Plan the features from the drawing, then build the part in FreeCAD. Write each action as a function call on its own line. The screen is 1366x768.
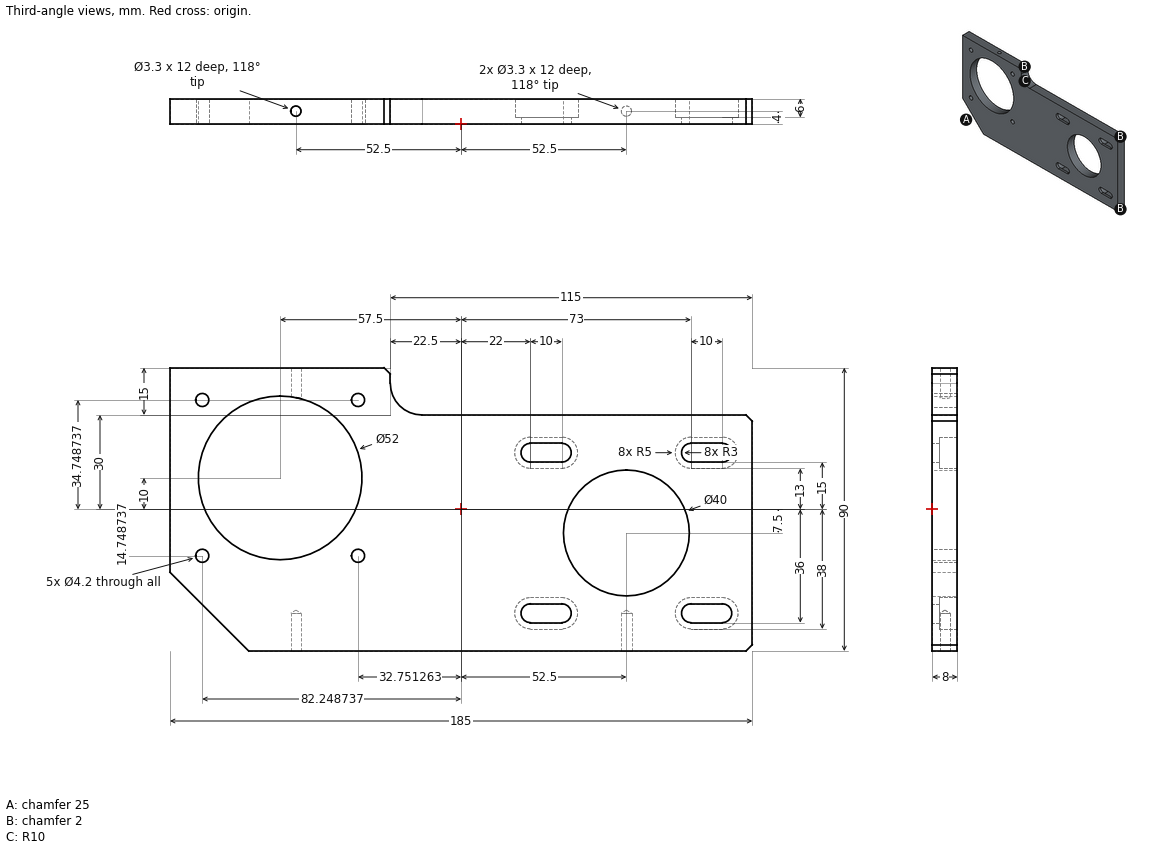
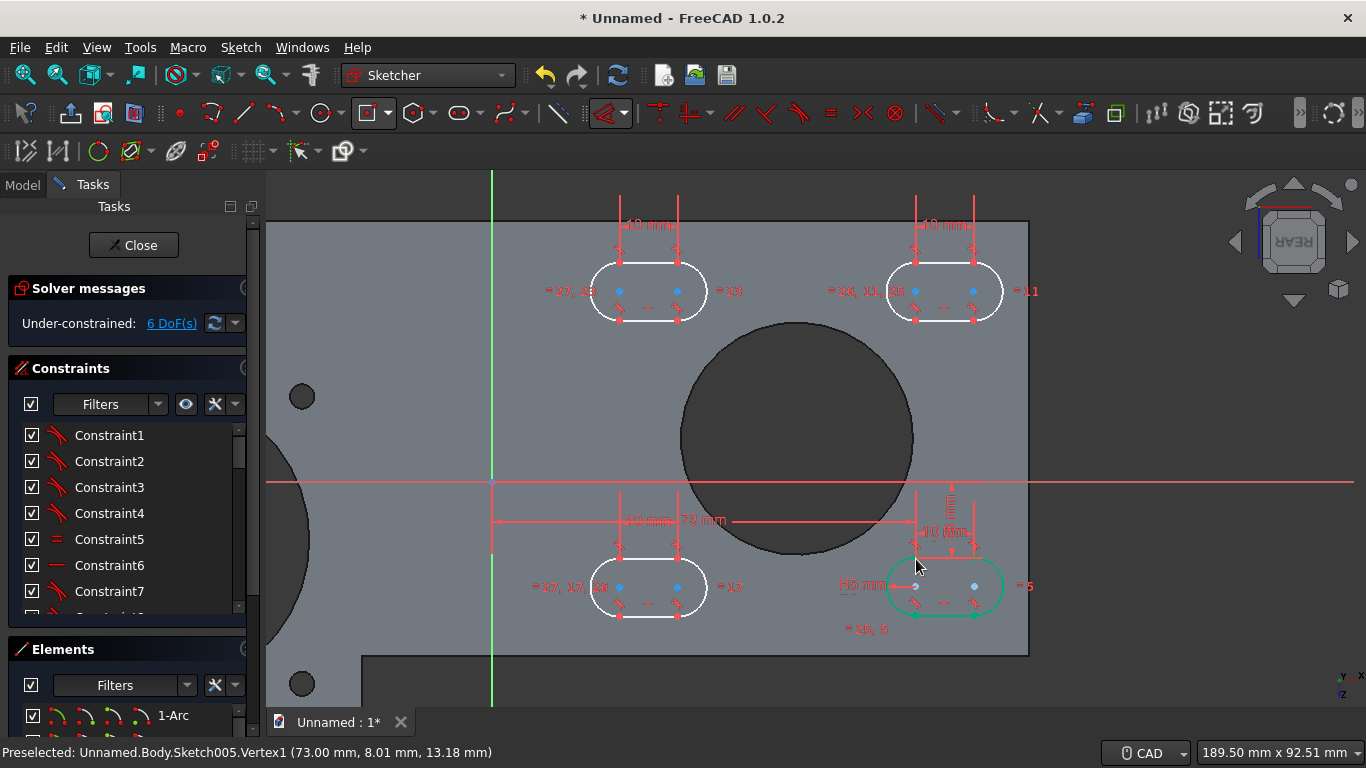
click(916, 263)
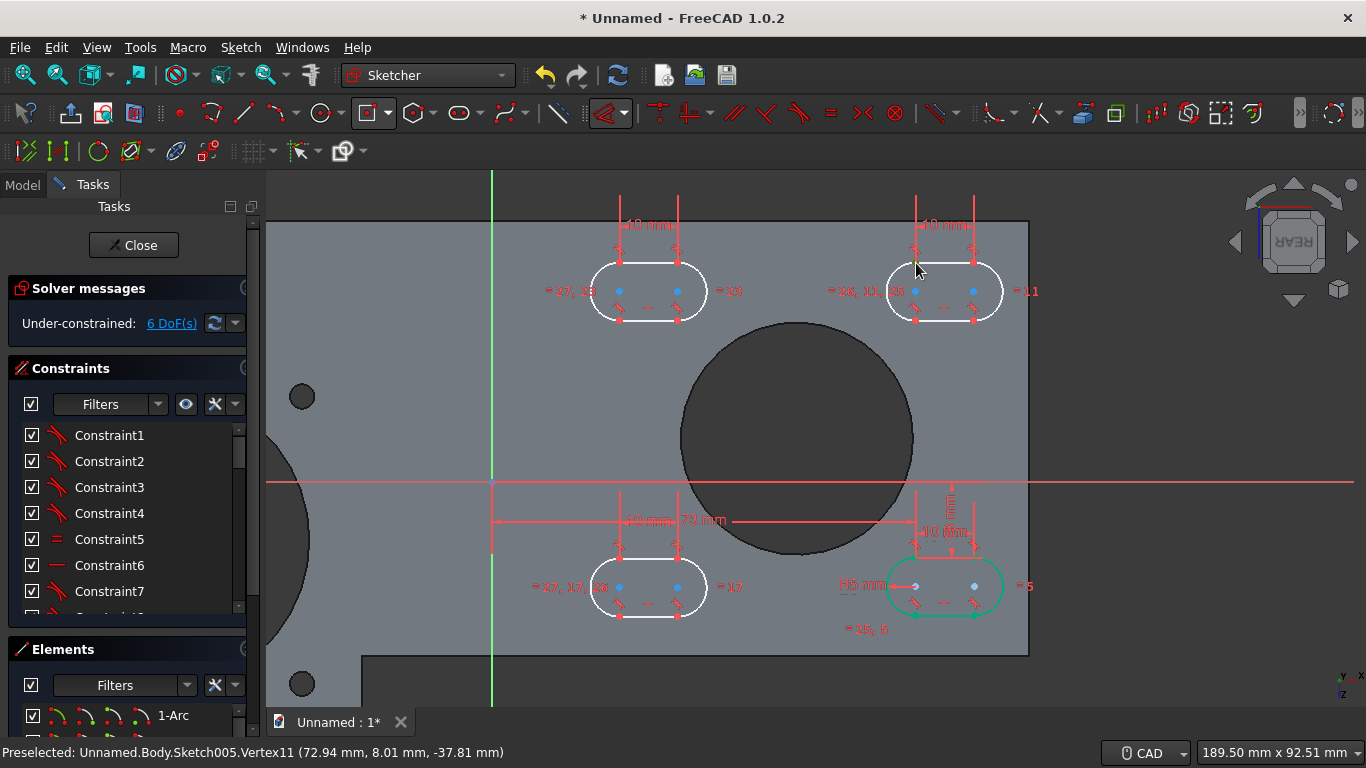
click(626, 114)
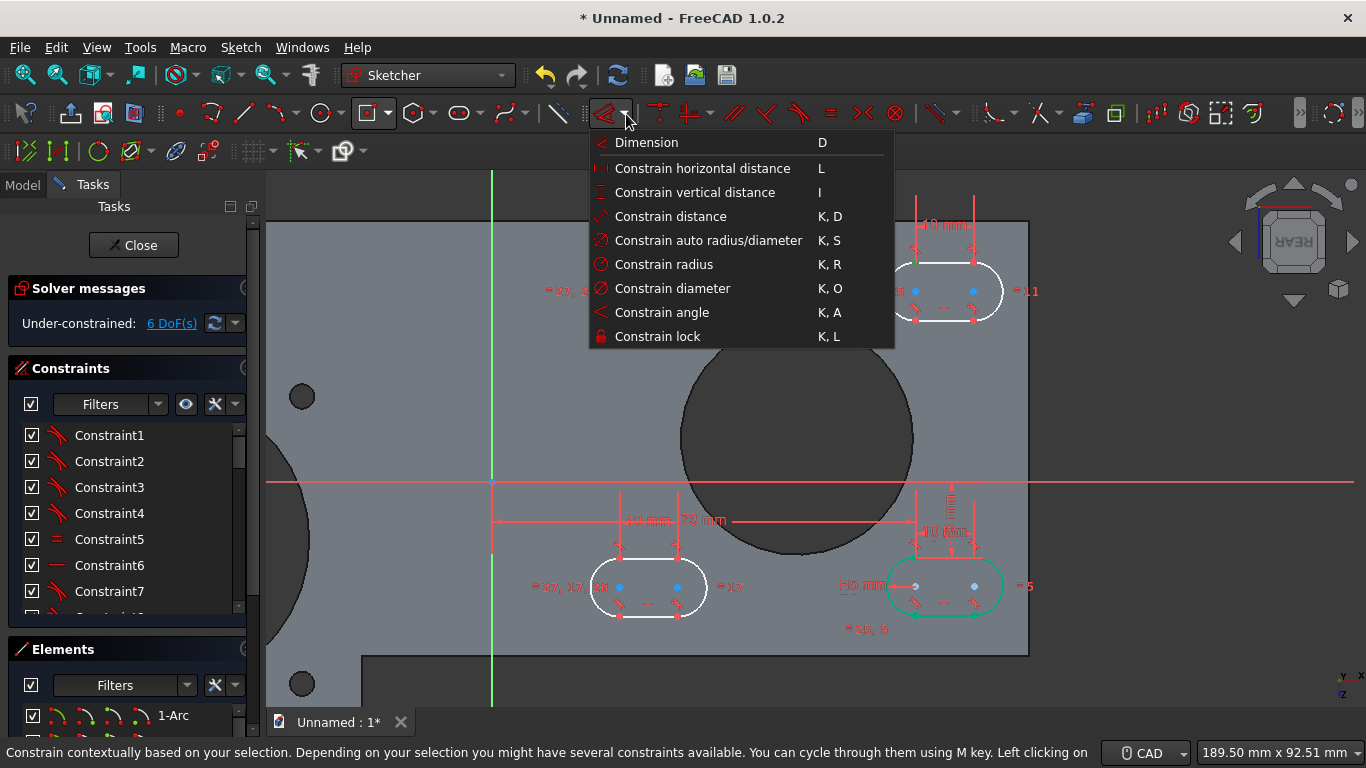
click(742, 168)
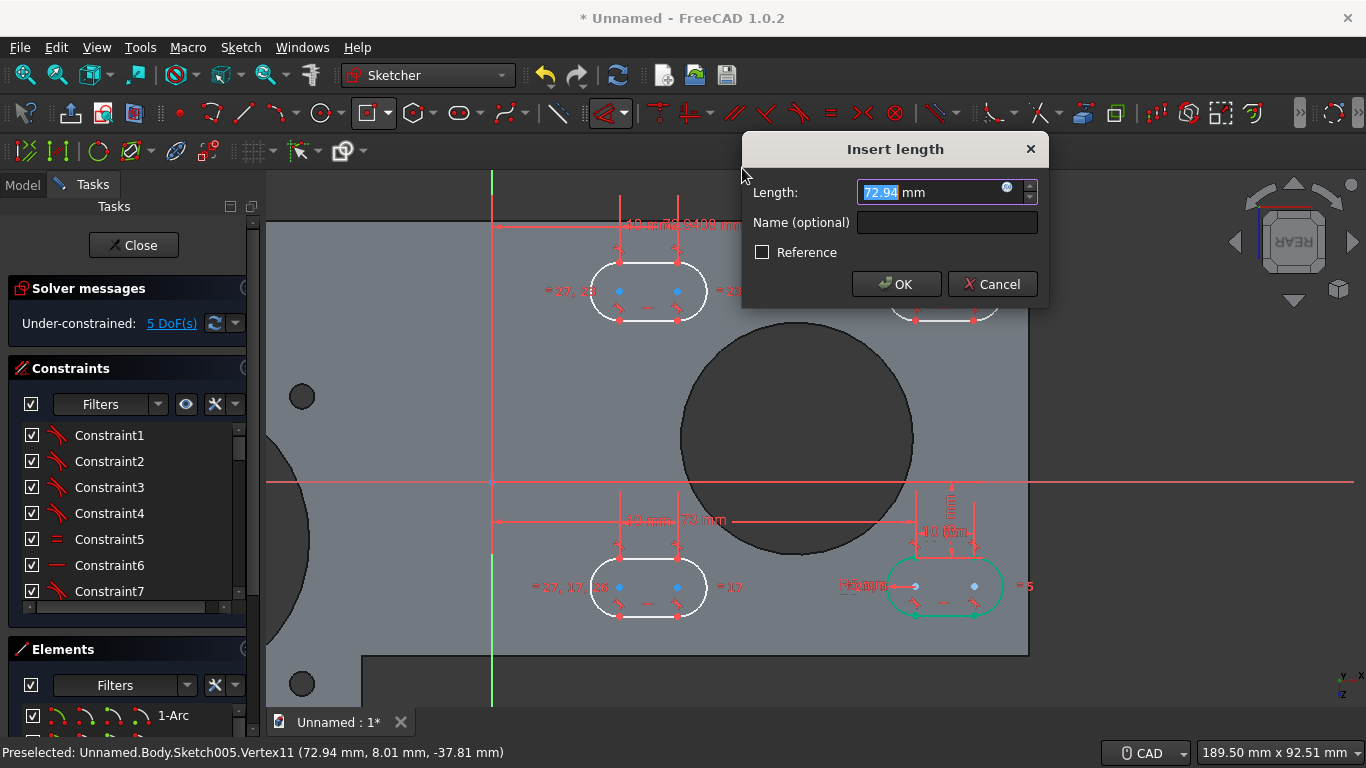
text(73)
key(Return)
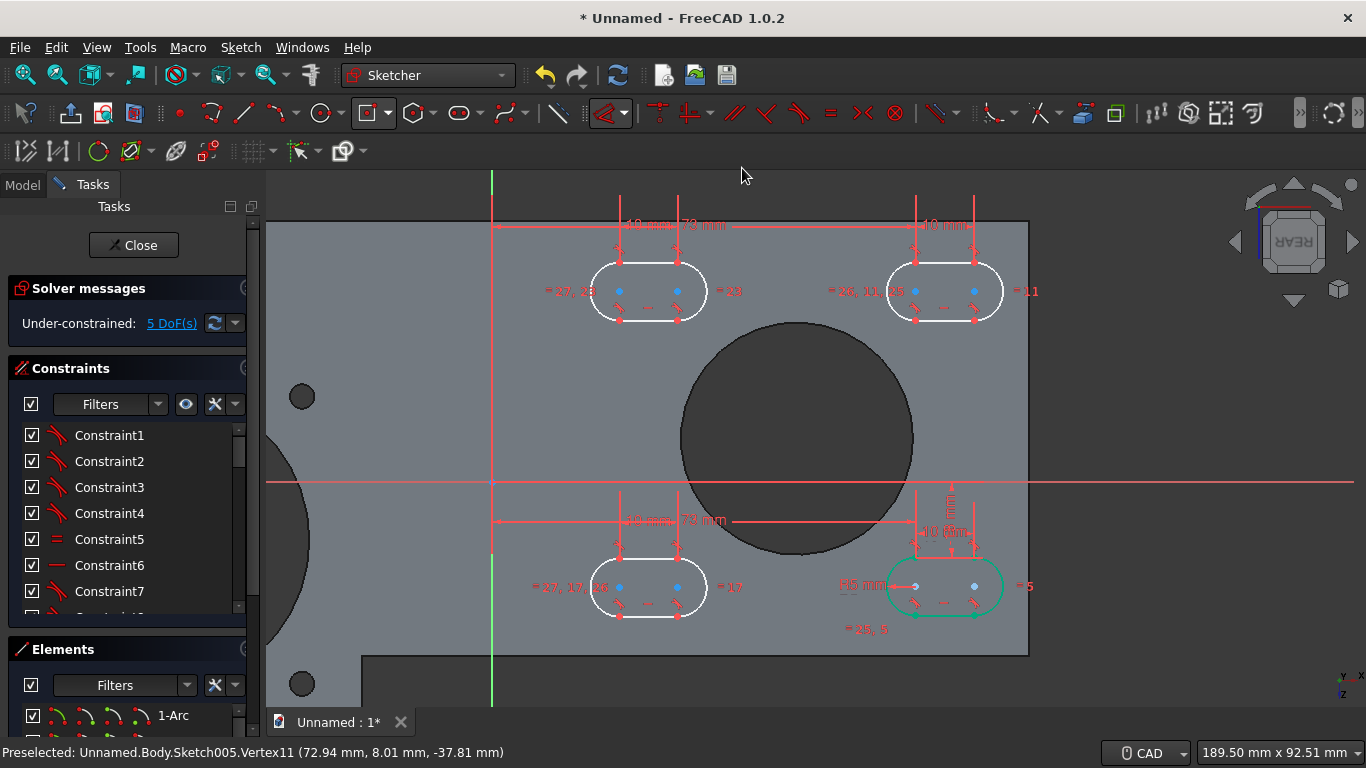
click(916, 263)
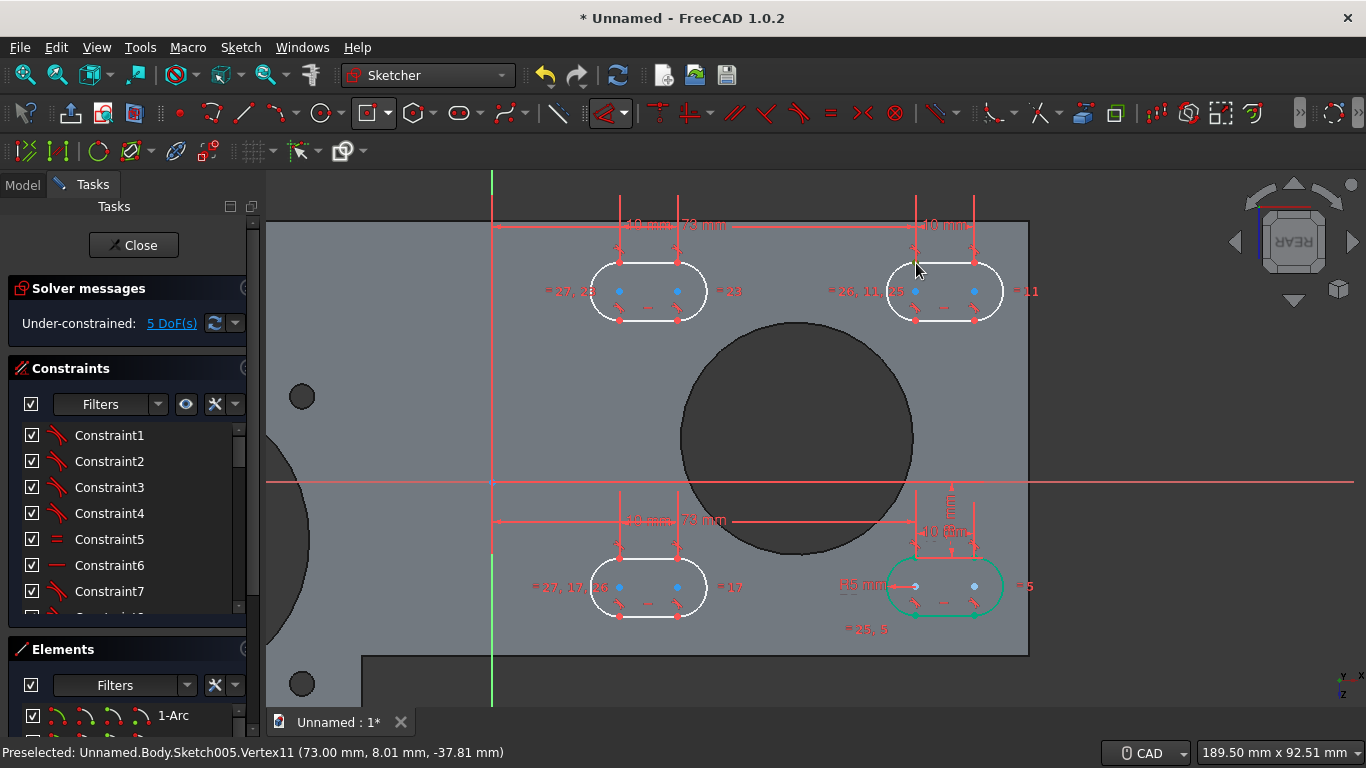
key(i)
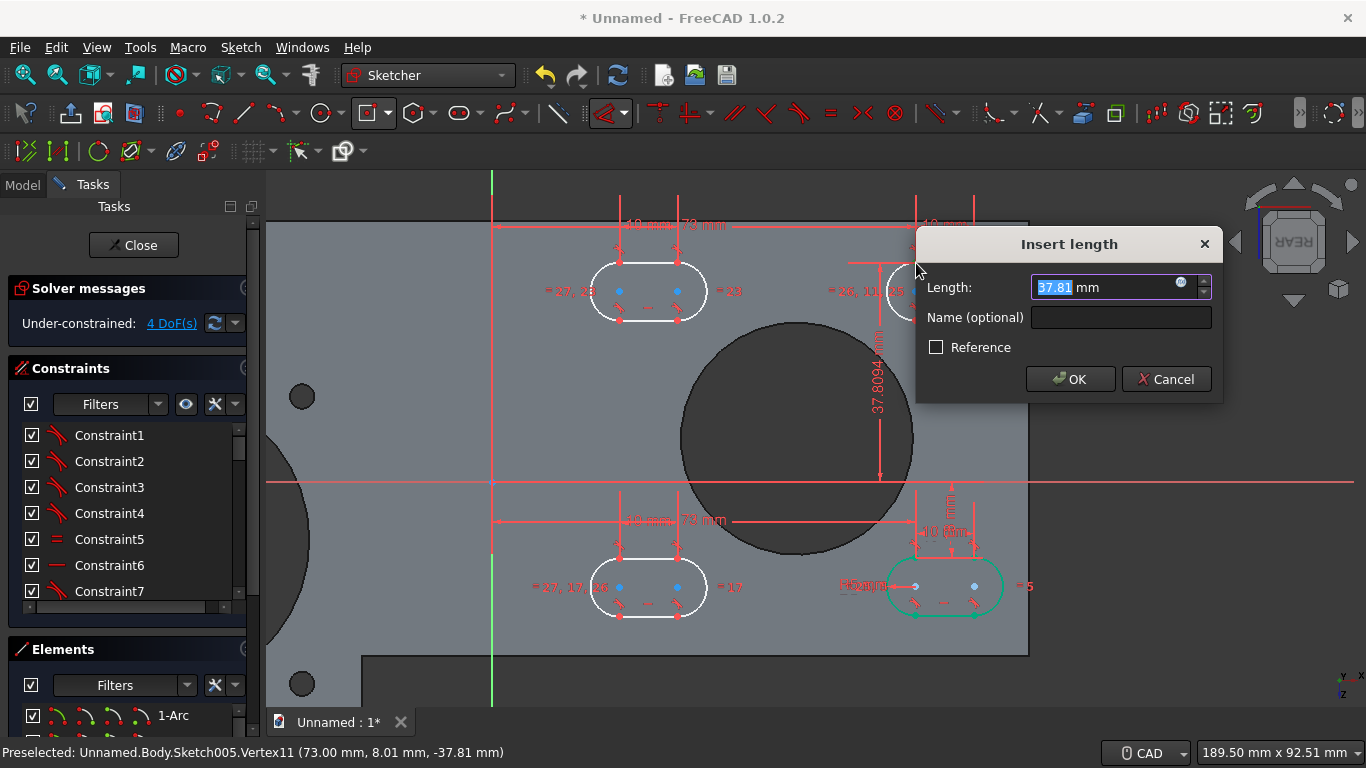
text(38)
key(Return)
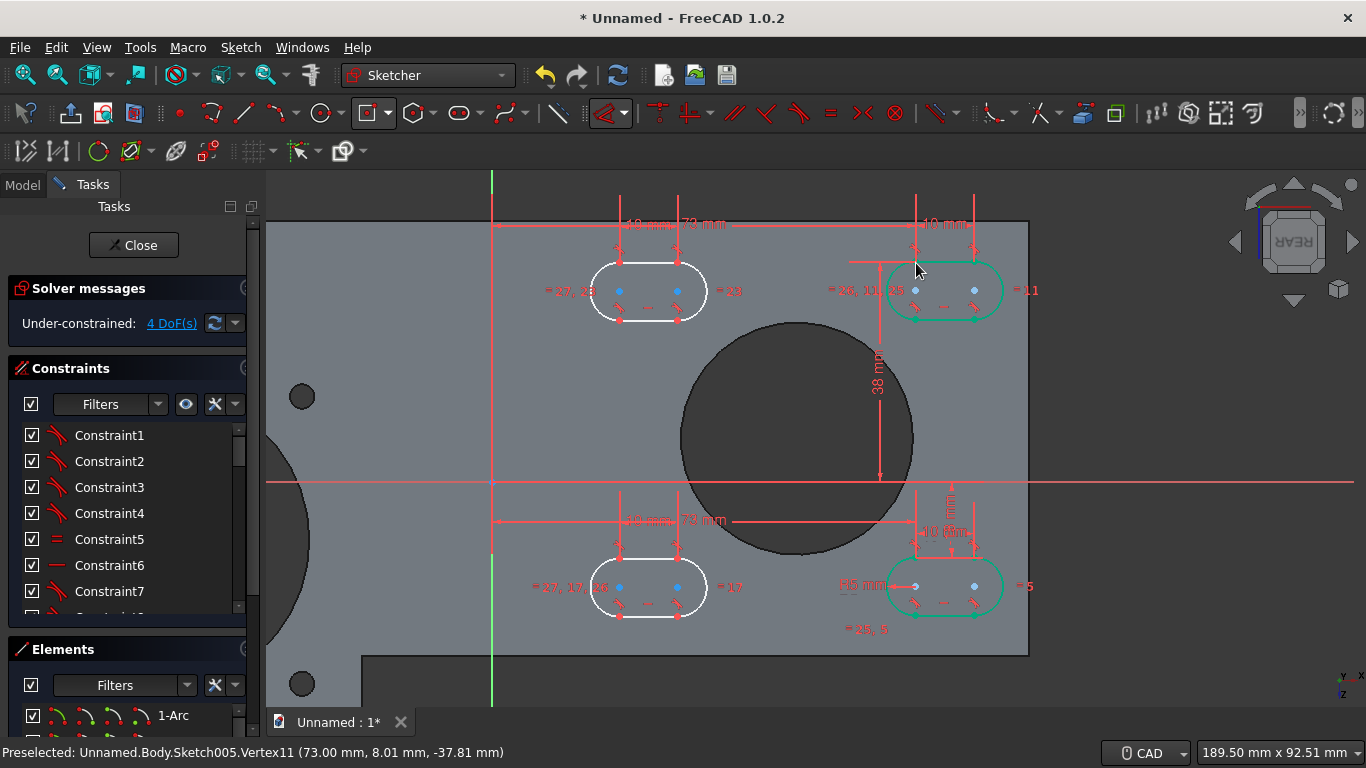
click(620, 559)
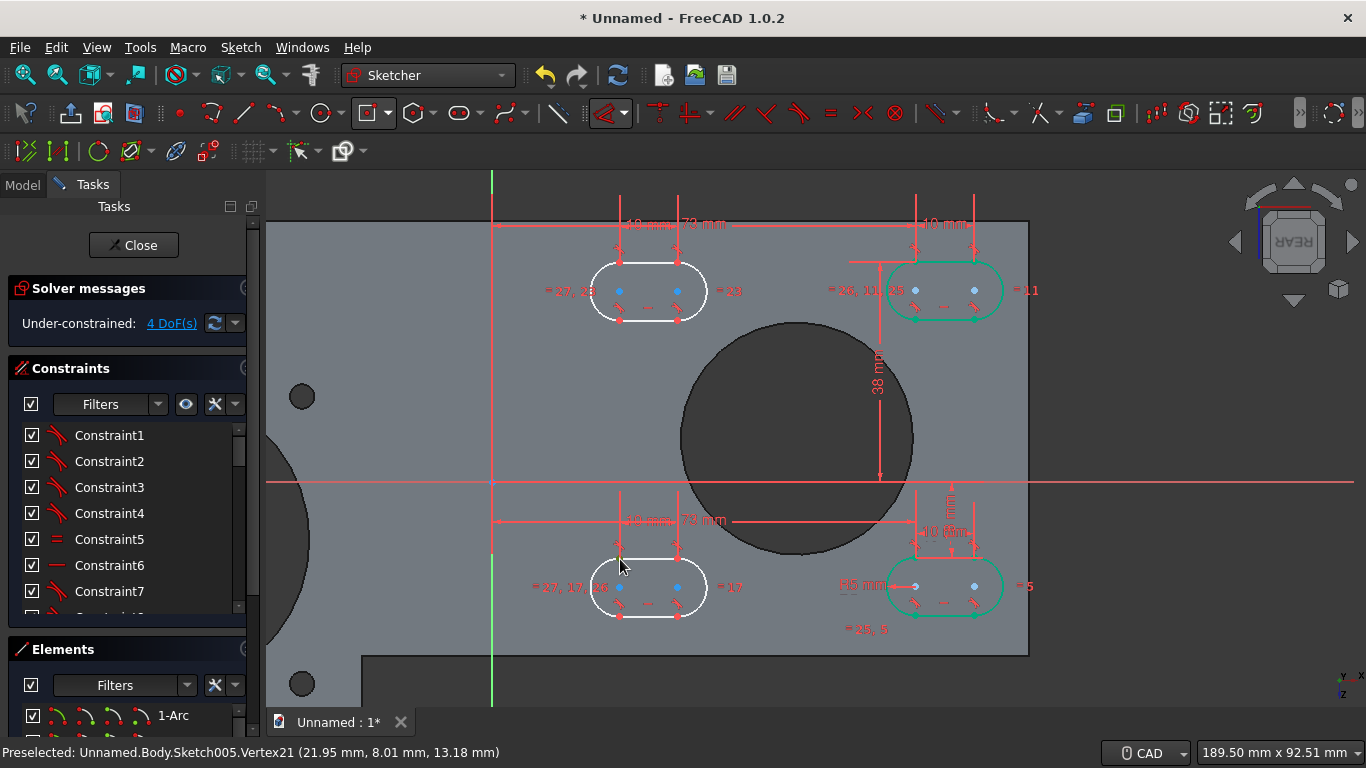
key(l)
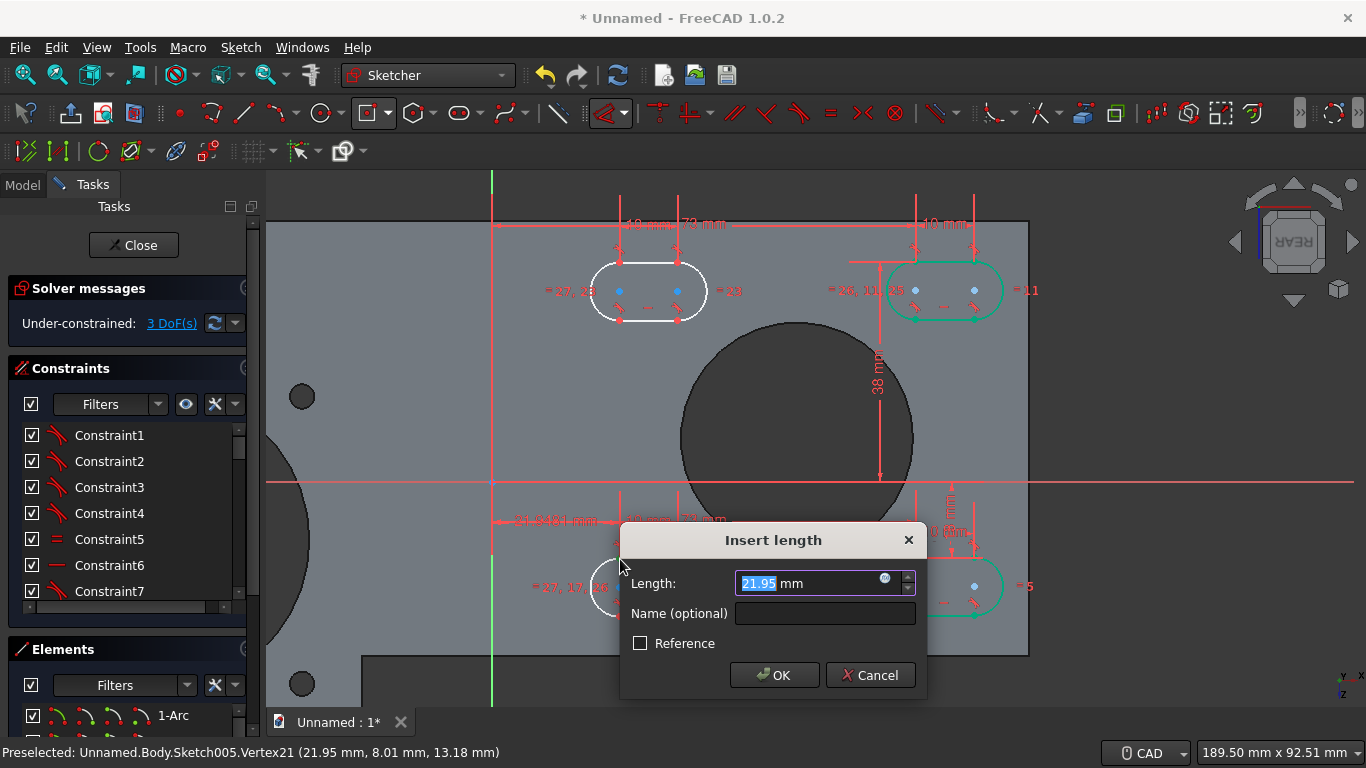
text(22)
key(Return)